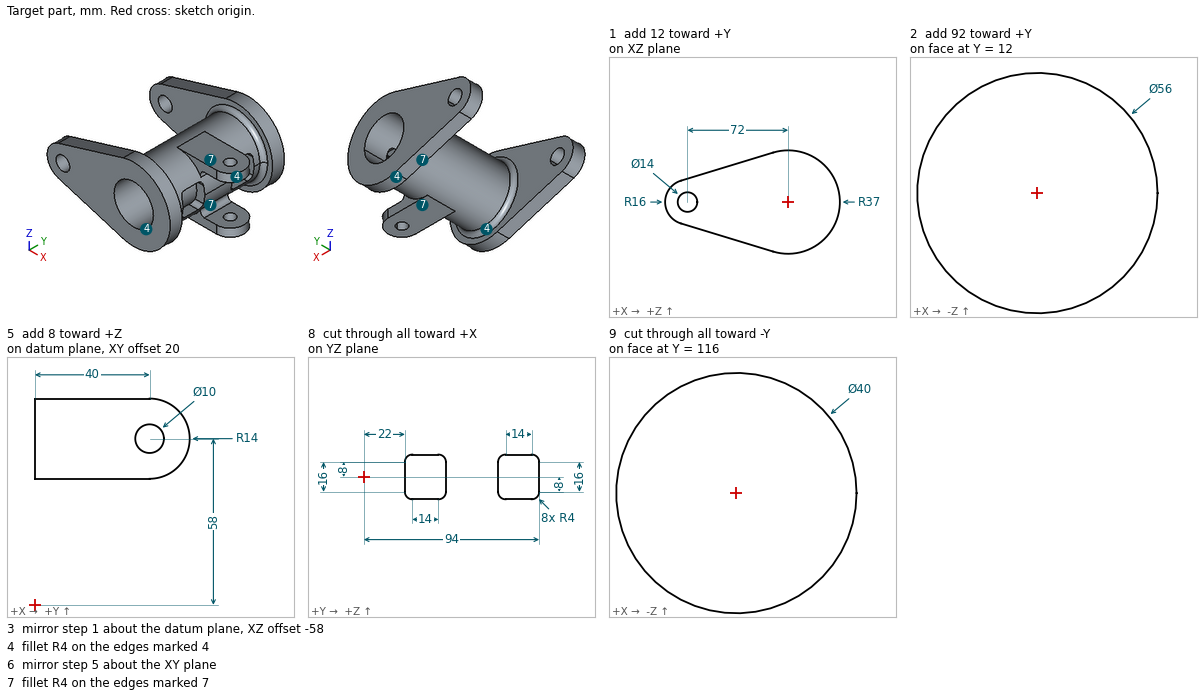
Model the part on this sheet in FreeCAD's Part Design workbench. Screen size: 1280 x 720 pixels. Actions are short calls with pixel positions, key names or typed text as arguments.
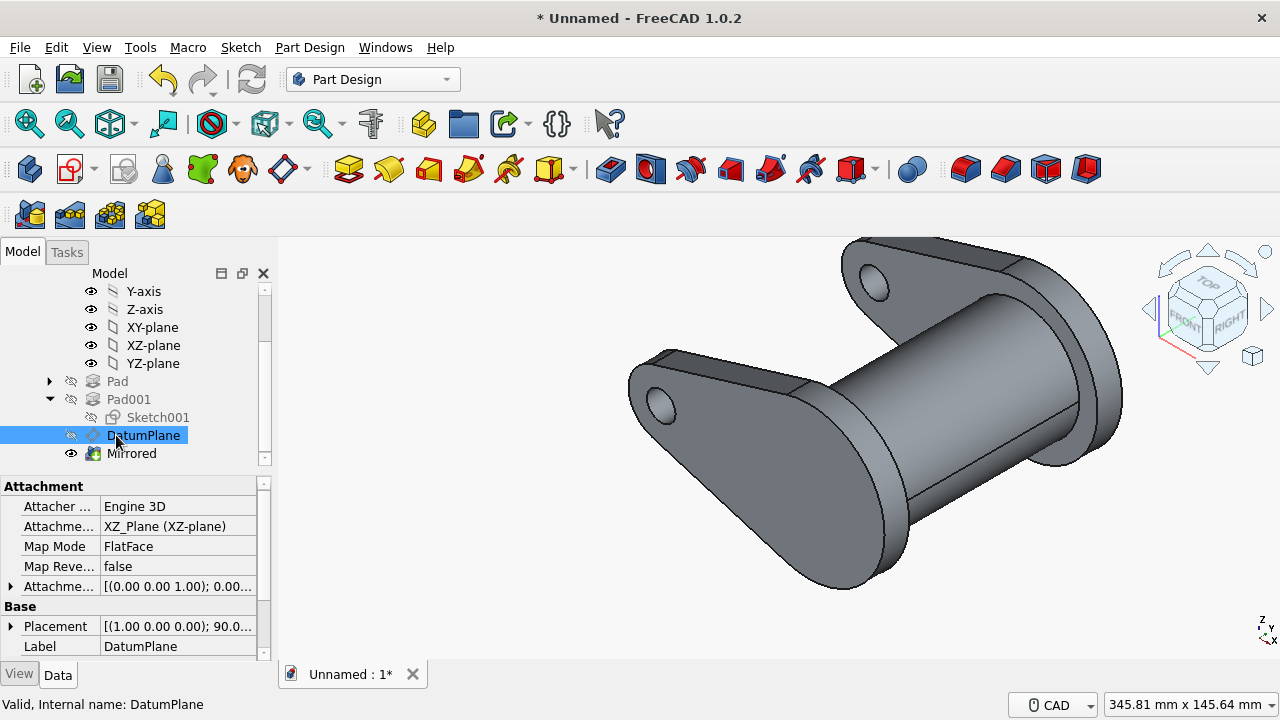
click(30, 124)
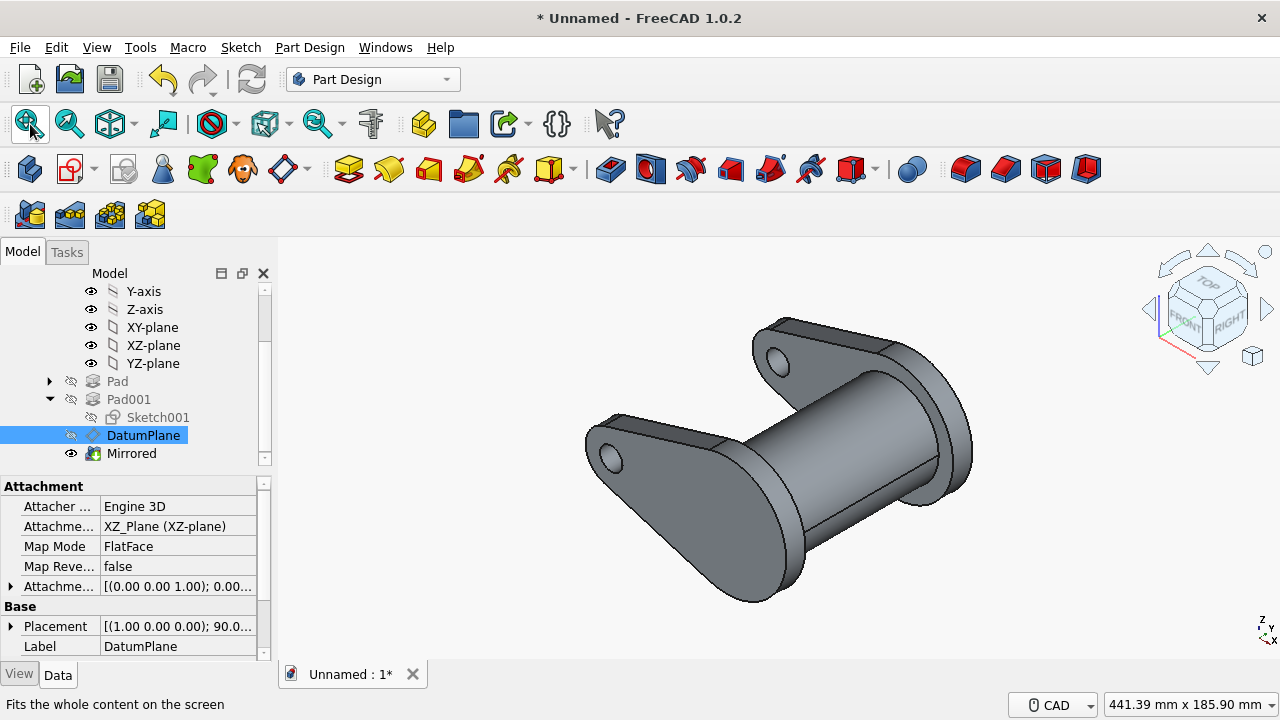
key(2)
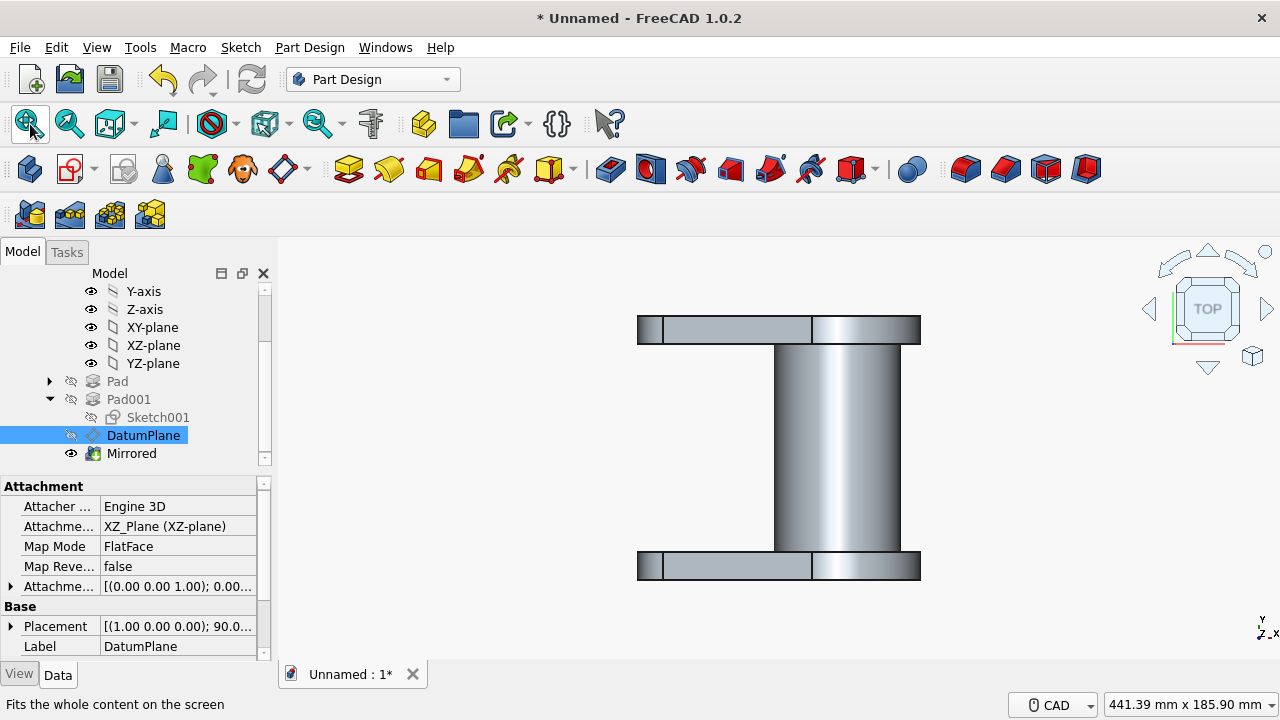
key(1)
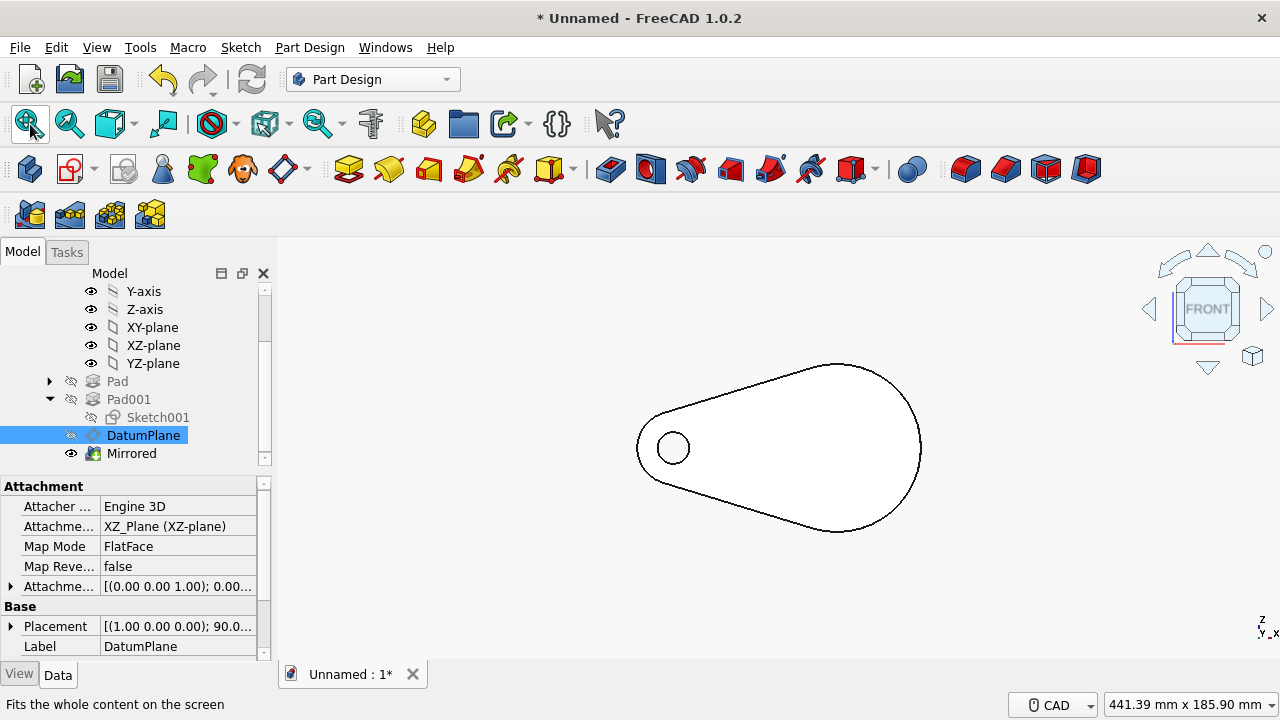
key(v)
key(f)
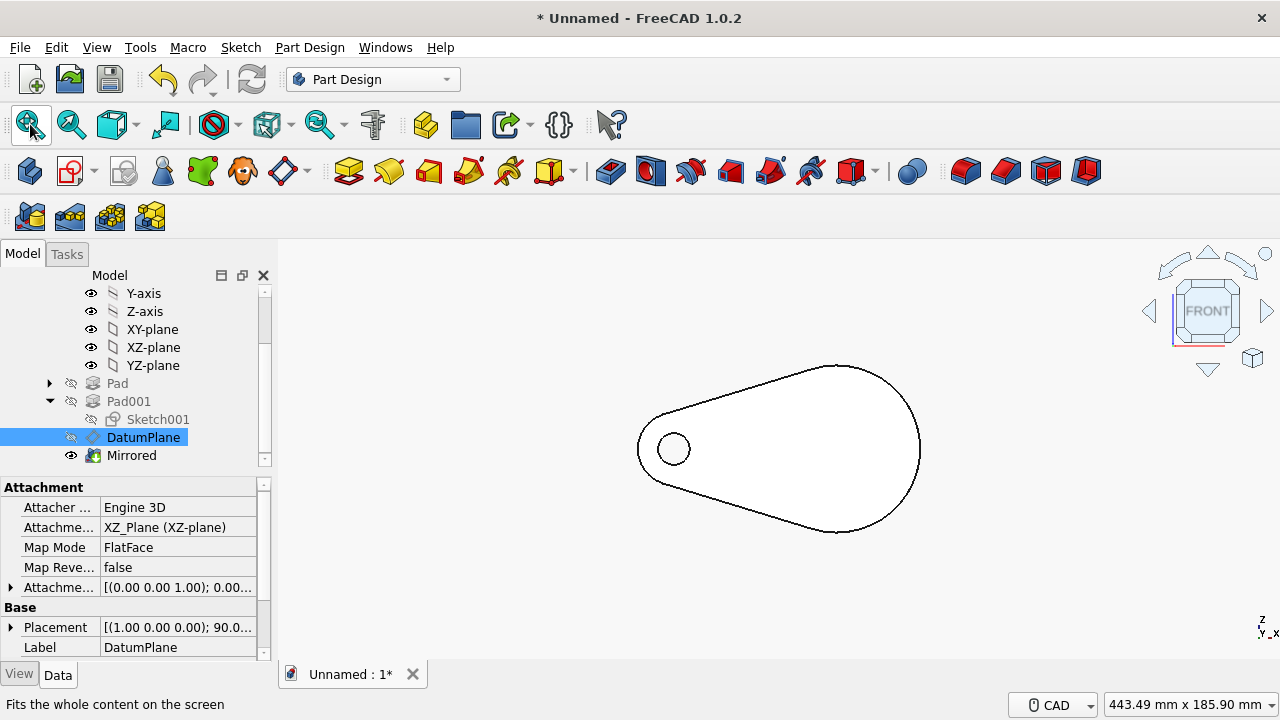
key(3)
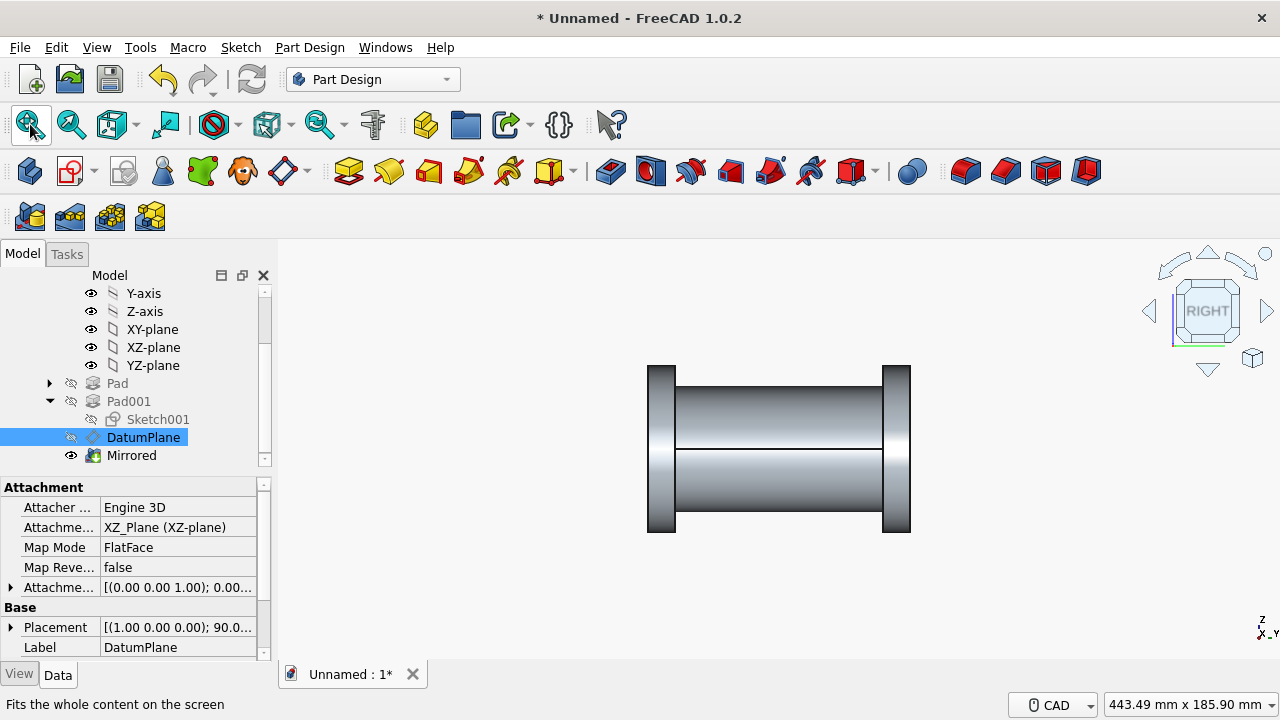
click(32, 126)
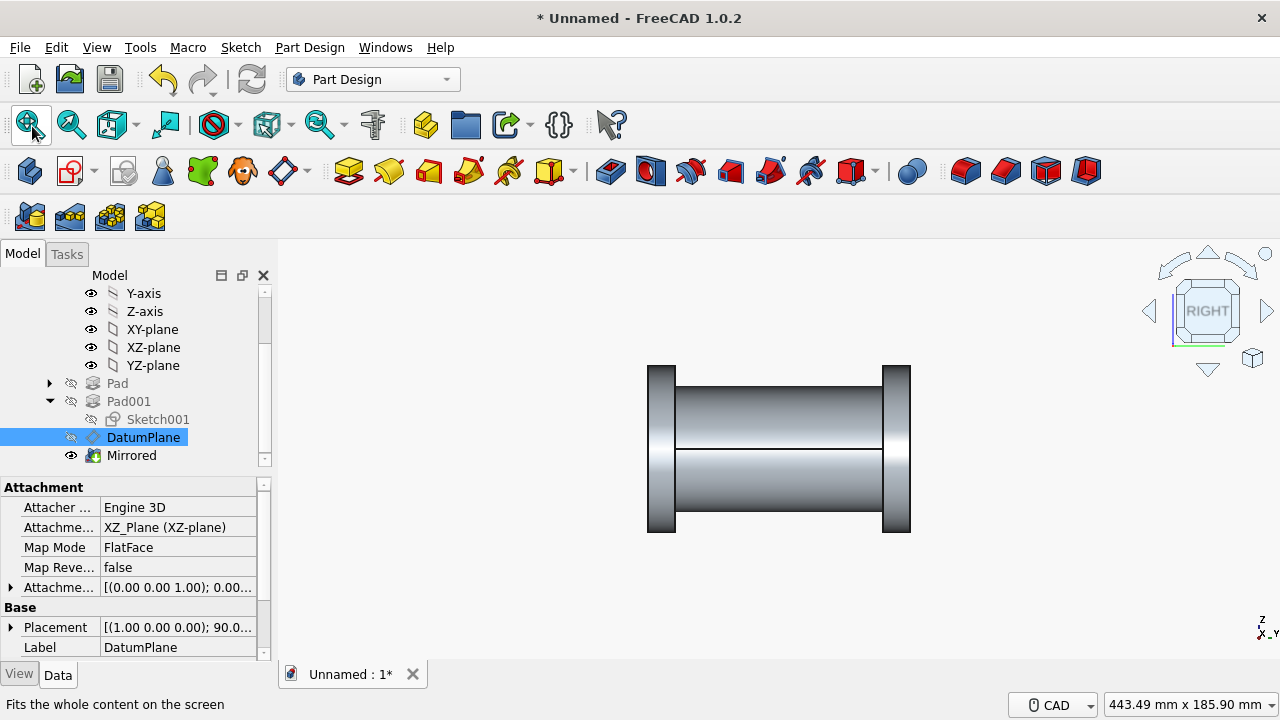
key(5)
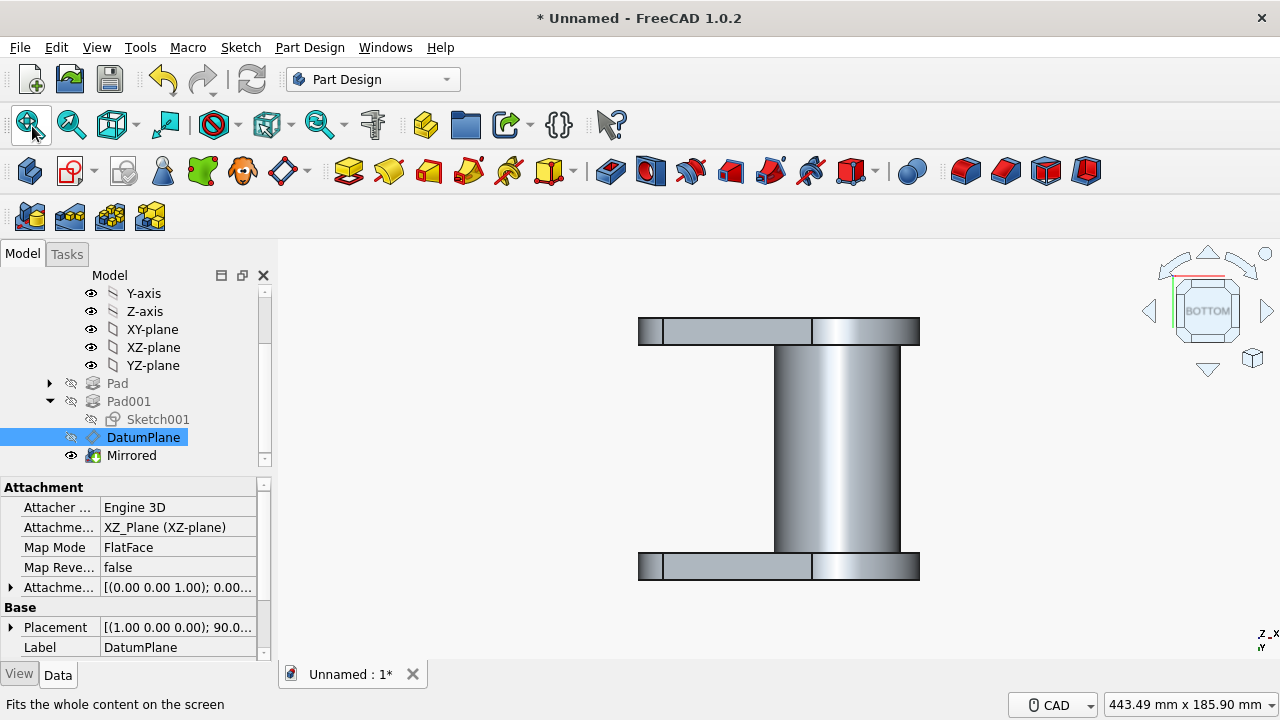
key(4)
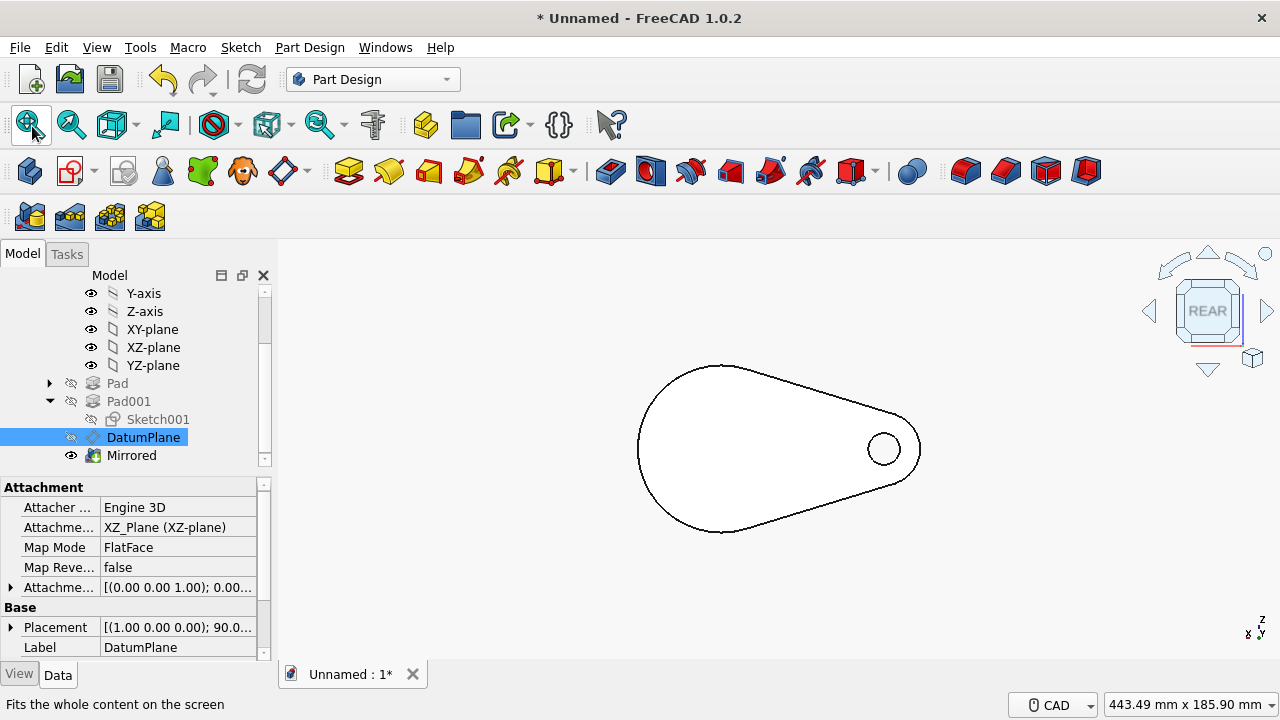
click(32, 126)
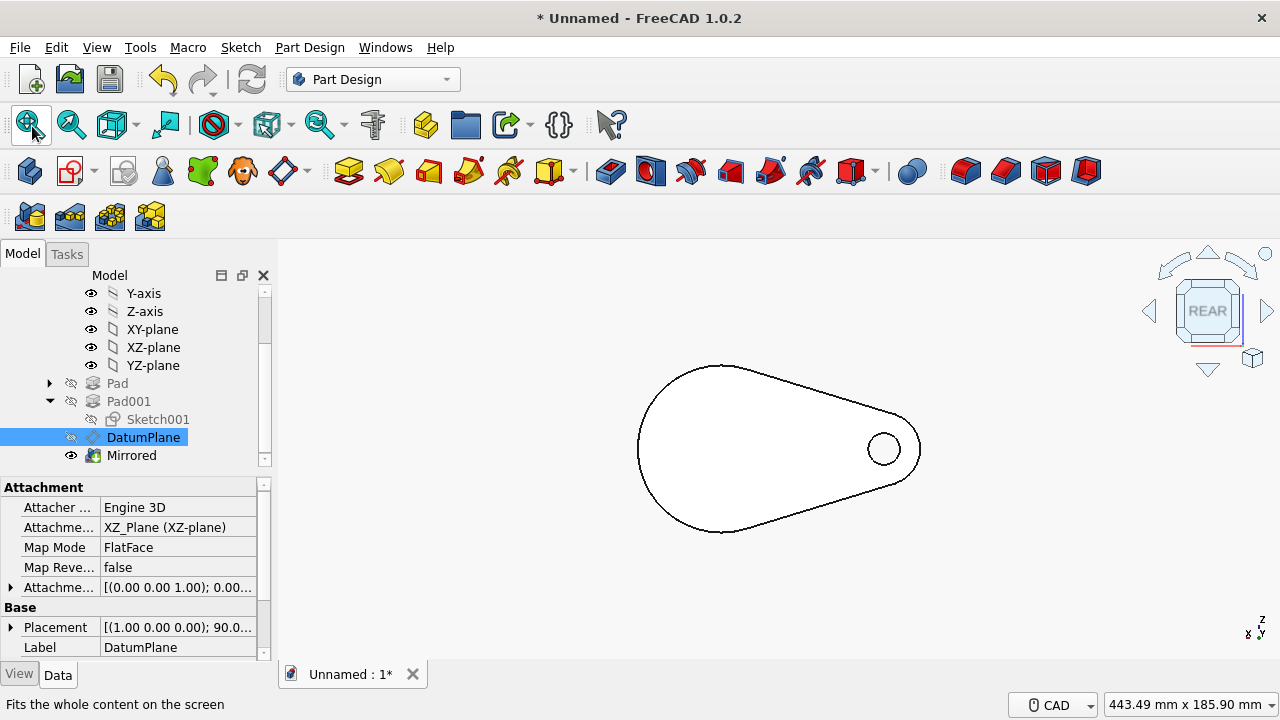
key(6)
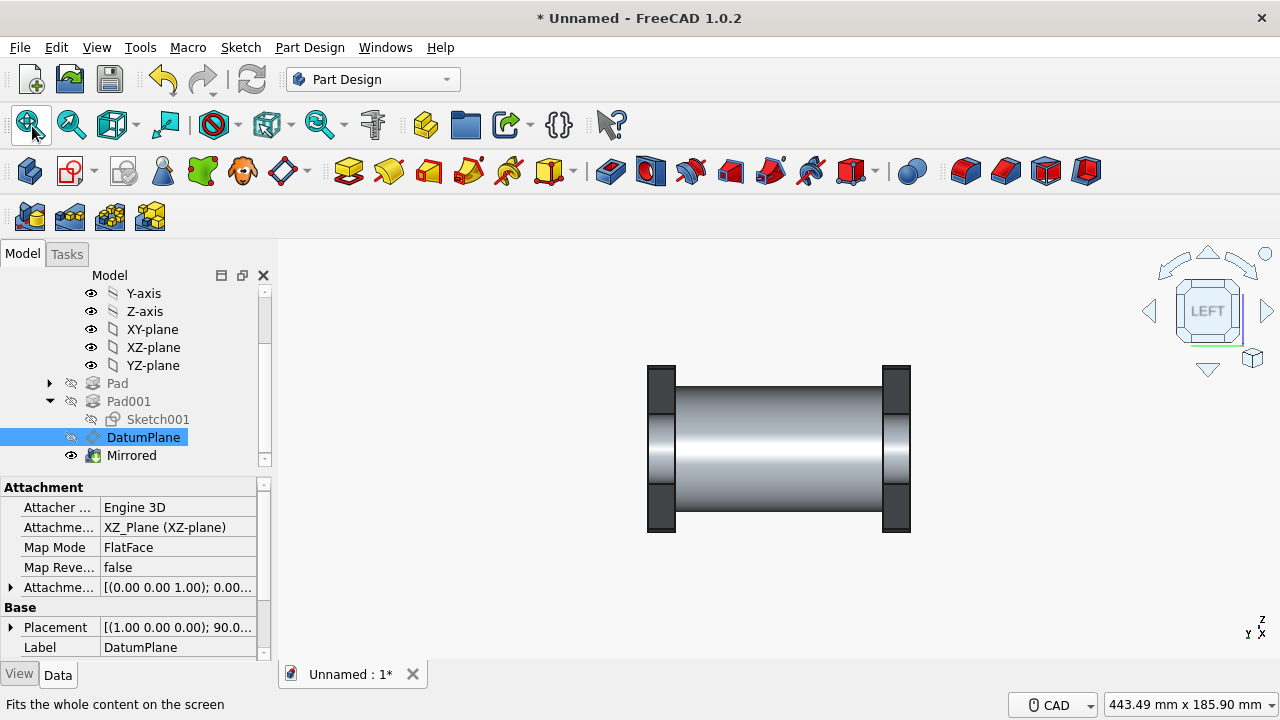
click(32, 126)